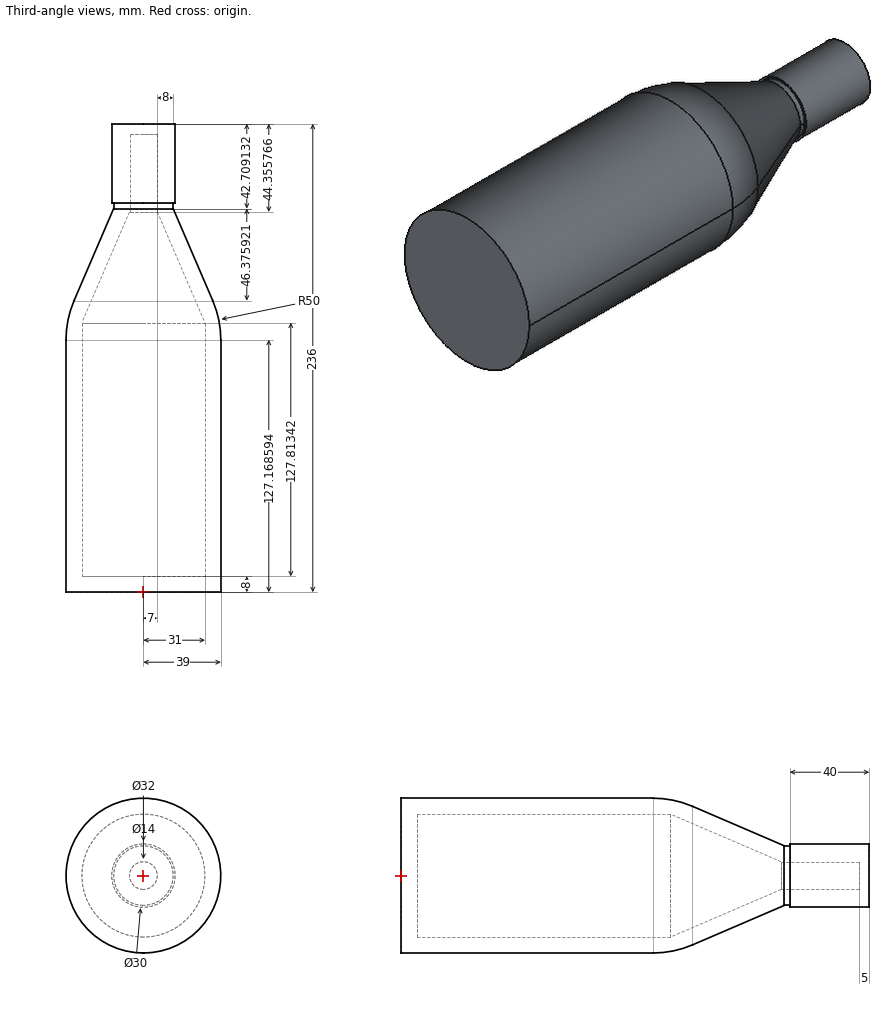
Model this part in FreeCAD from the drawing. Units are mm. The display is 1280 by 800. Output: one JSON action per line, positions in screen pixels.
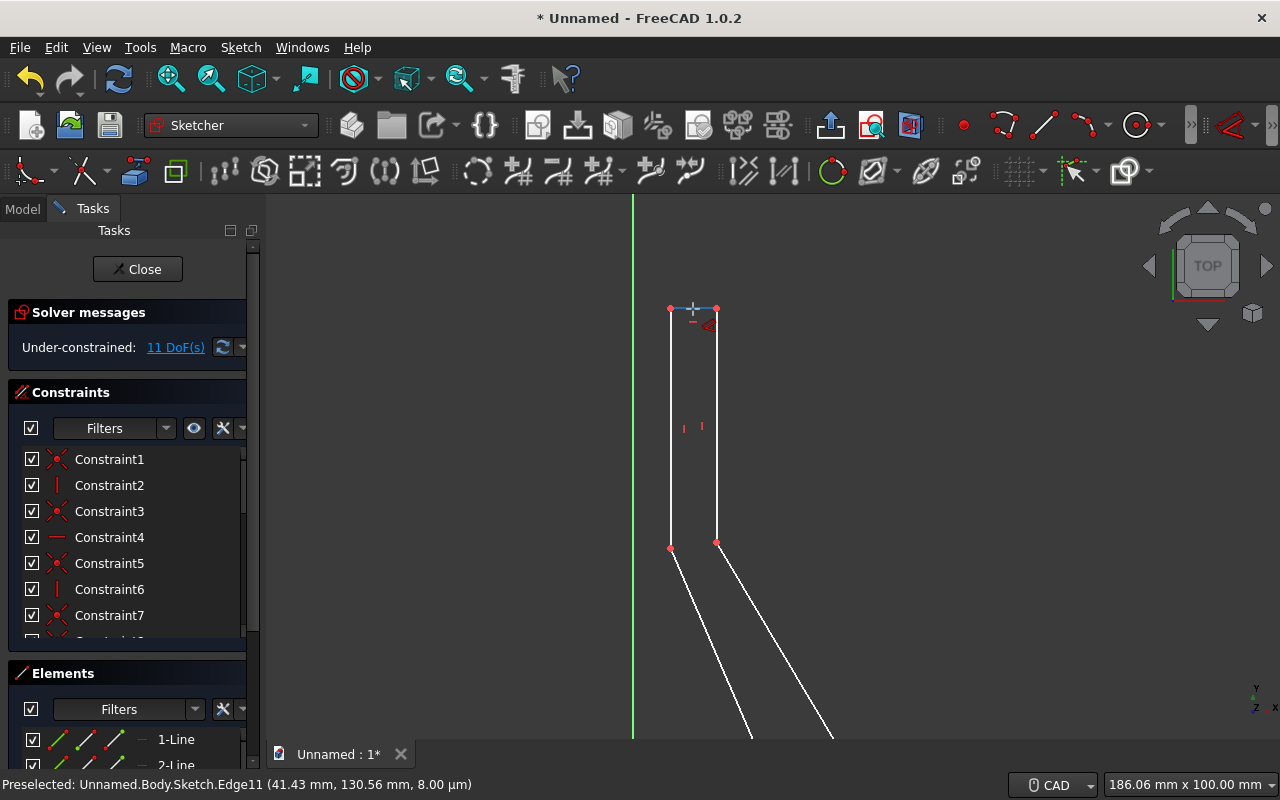
{"action": "left_click", "coordinate": [694, 308]}
{"action": "left_click", "coordinate": [694, 274]}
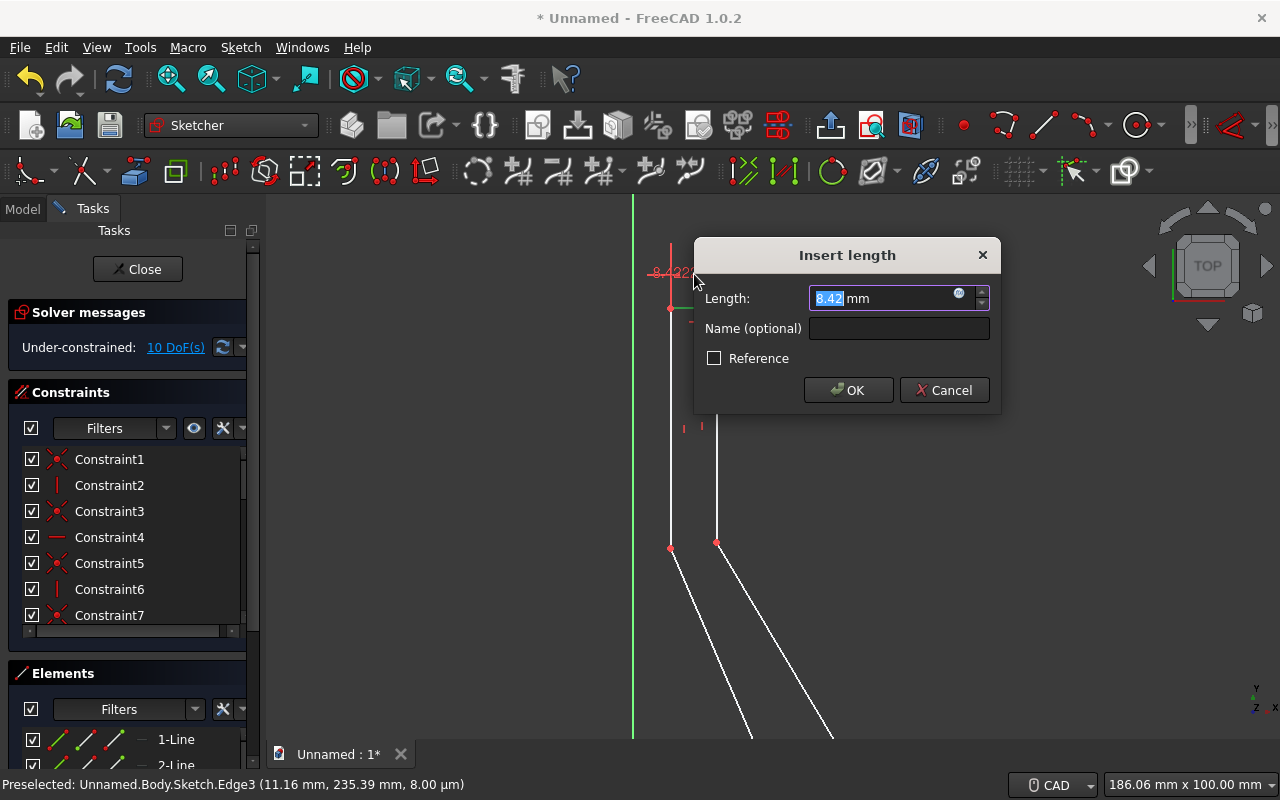
{"action": "type", "text": "8"}
{"action": "key", "text": "Return"}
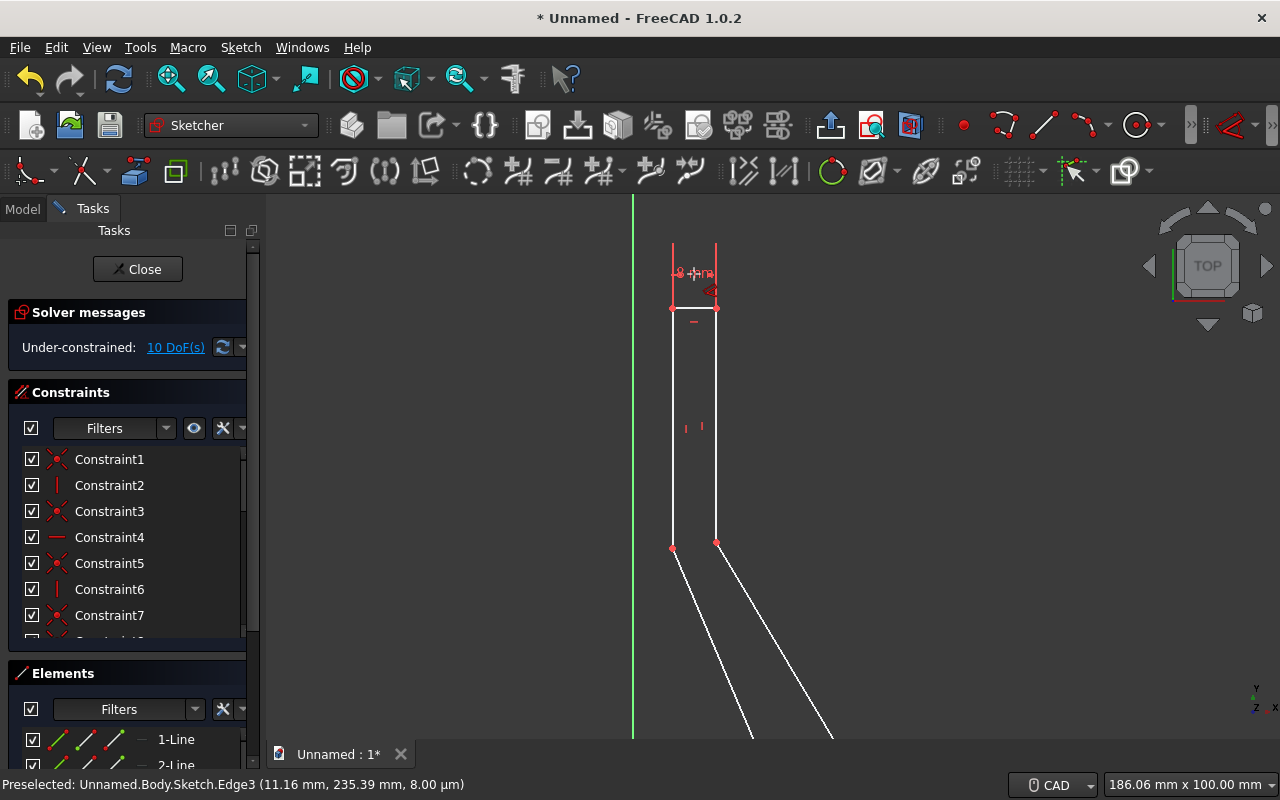
{"action": "scroll", "coordinate": [693, 309], "scroll_direction": "down", "scroll_amount": 7}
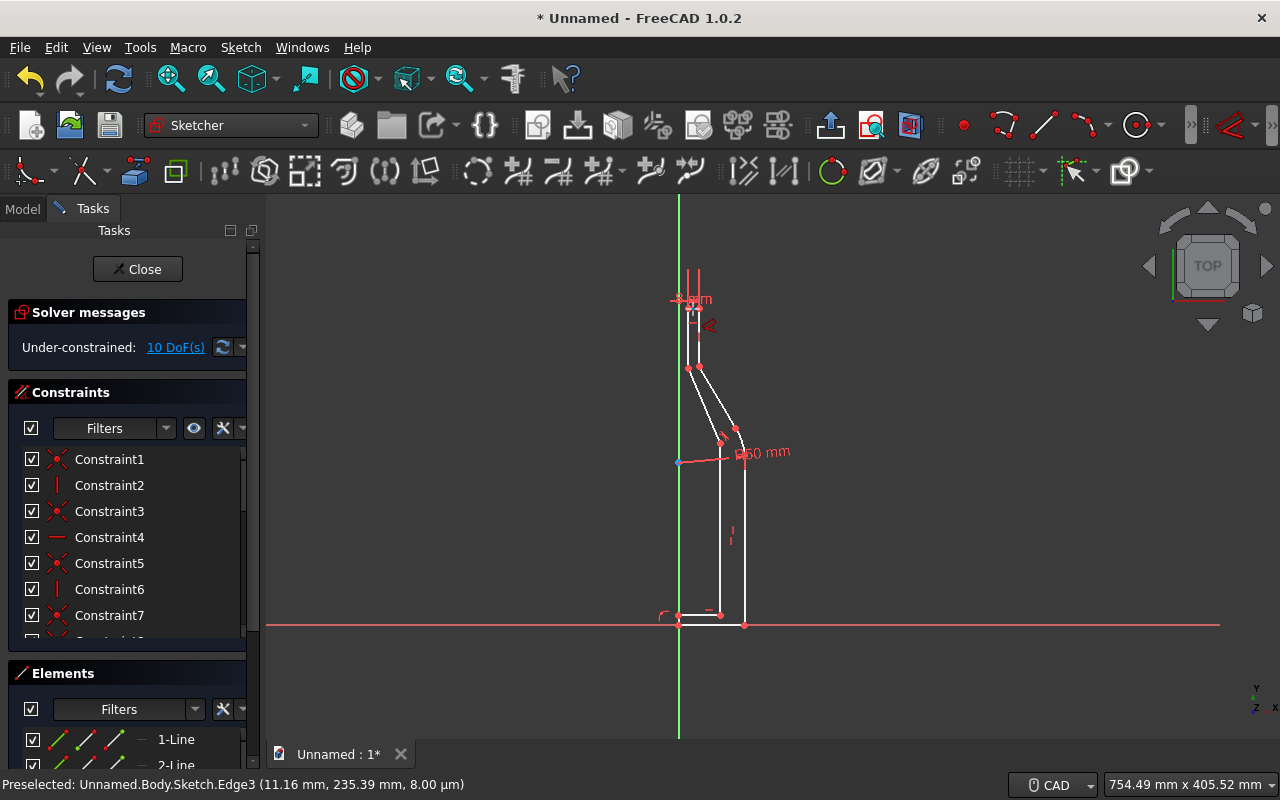
{"action": "scroll", "coordinate": [679, 618], "scroll_direction": "up", "scroll_amount": 8}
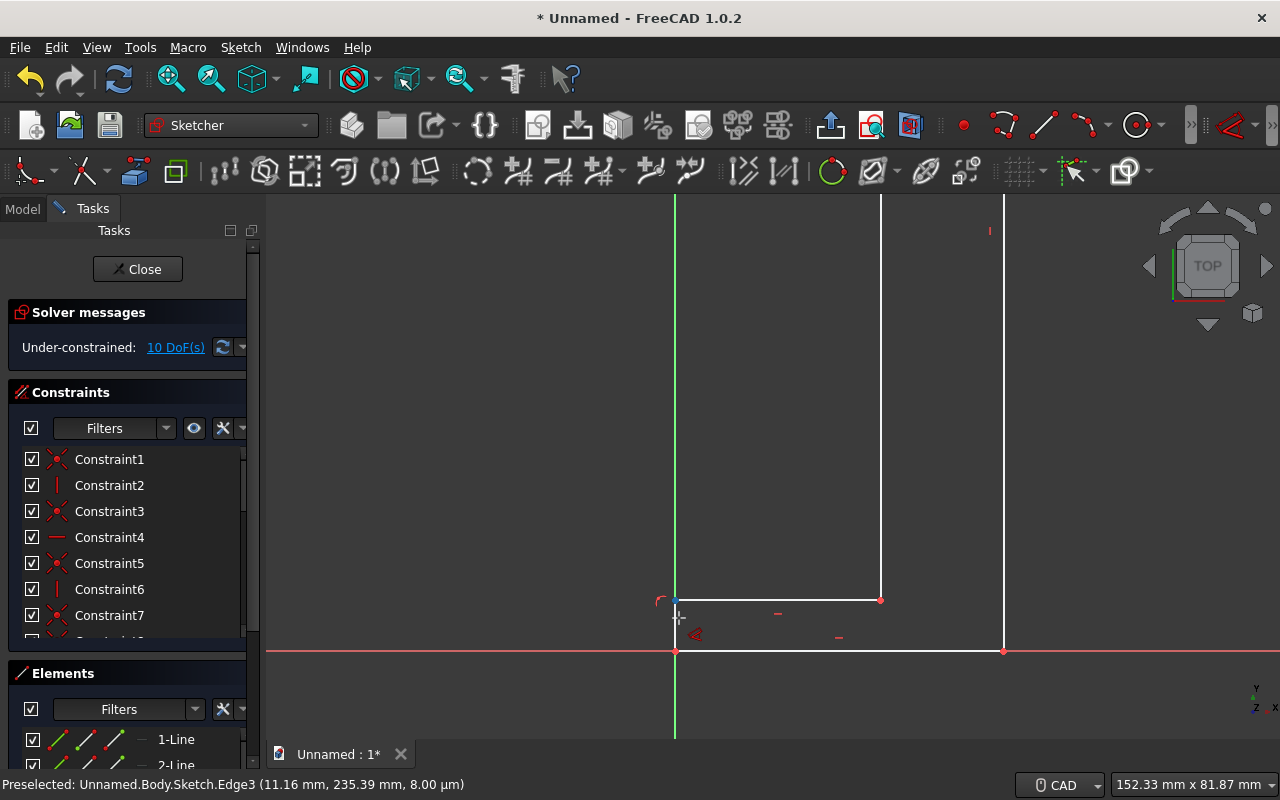
{"action": "left_click", "coordinate": [675, 615]}
{"action": "left_click", "coordinate": [641, 626]}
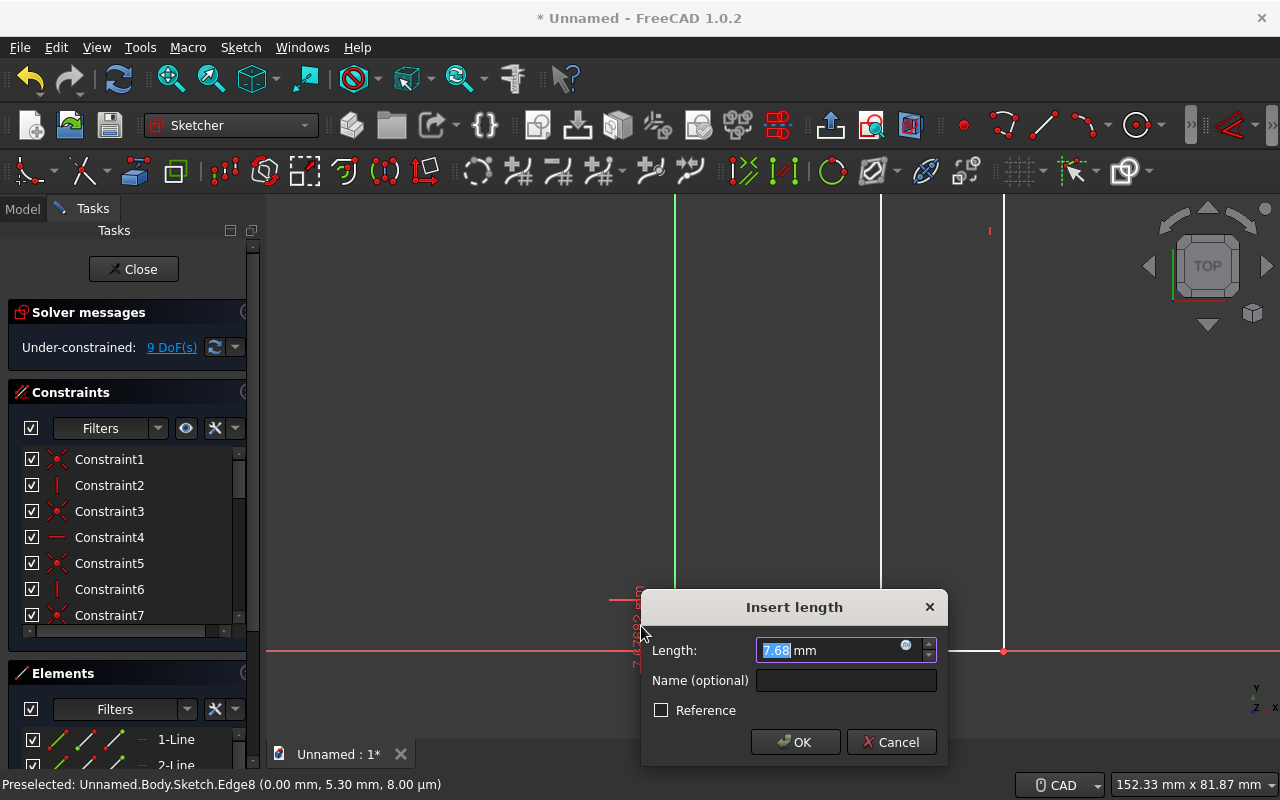
{"action": "type", "text": "8"}
{"action": "key", "text": "Return"}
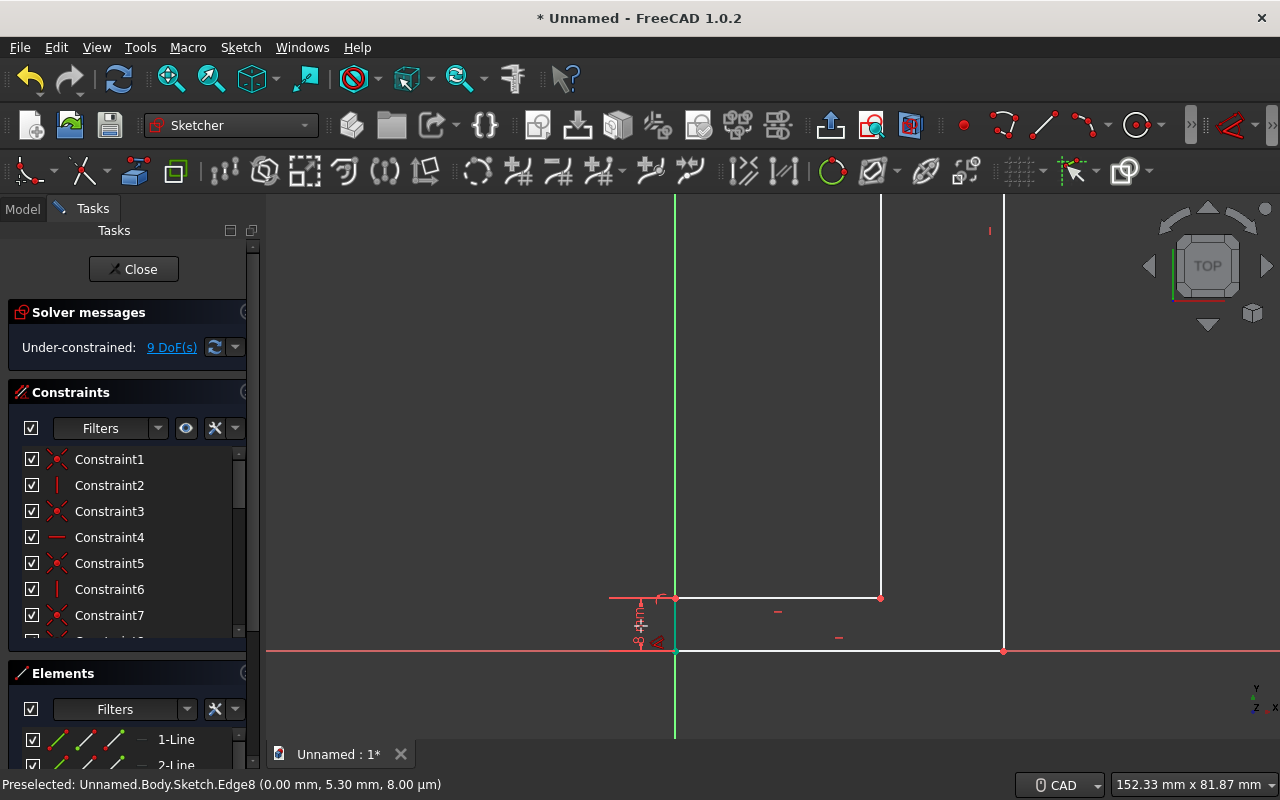
{"action": "scroll", "coordinate": [679, 618], "scroll_direction": "down", "scroll_amount": 8}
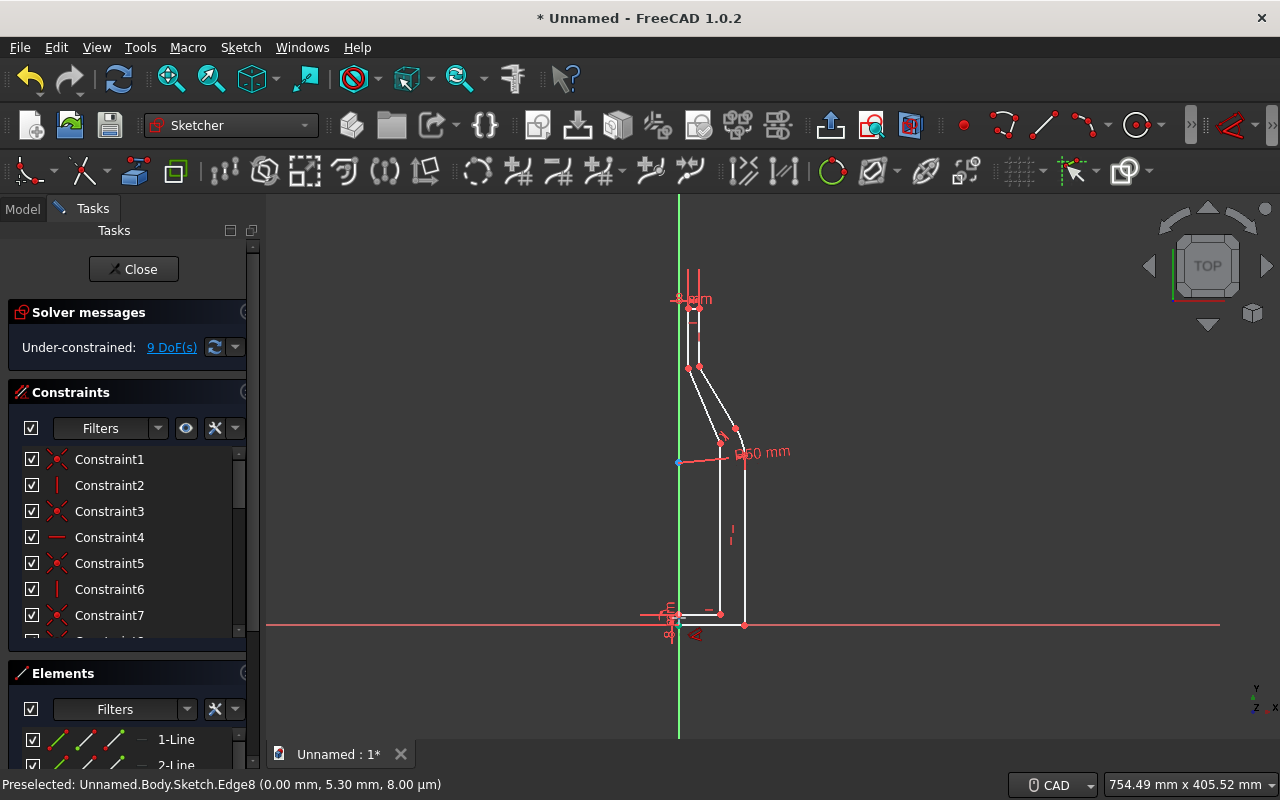
{"action": "scroll", "coordinate": [708, 615], "scroll_direction": "up", "scroll_amount": 2}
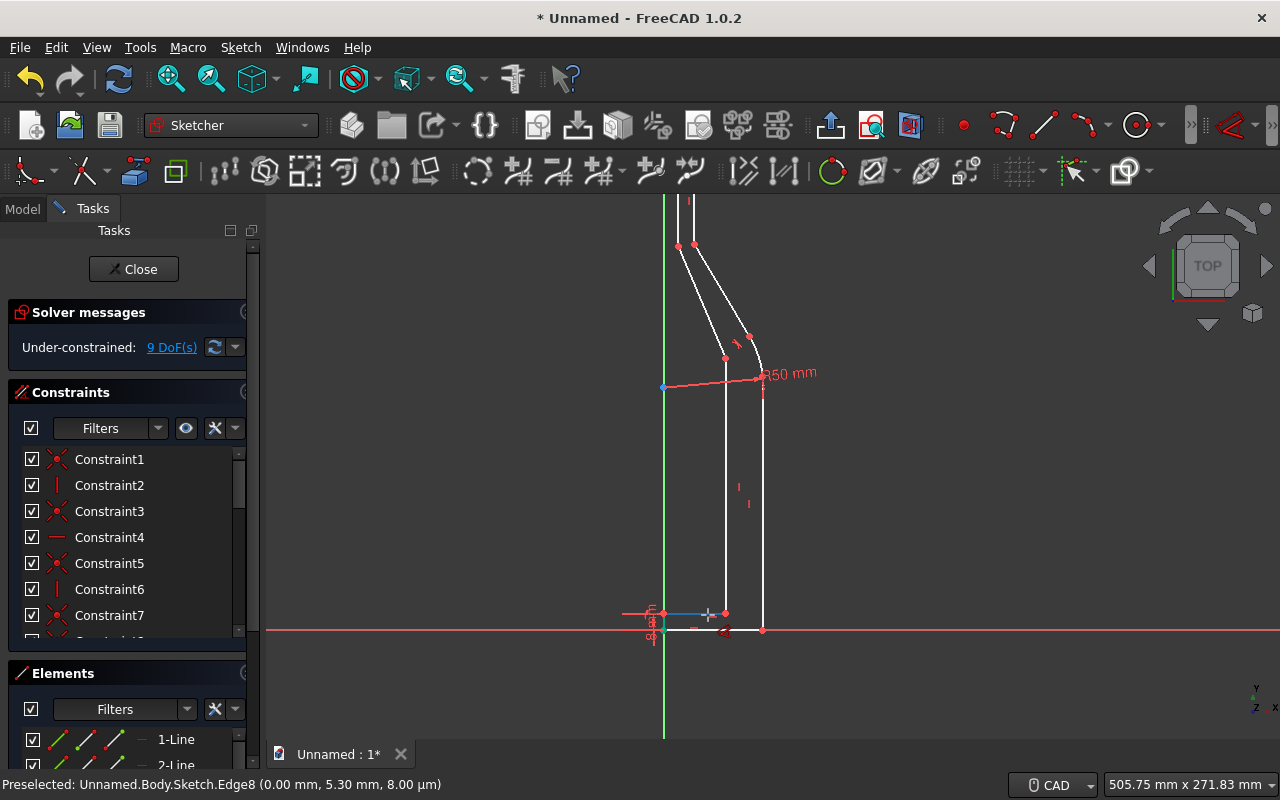
{"action": "left_click", "coordinate": [707, 614]}
{"action": "left_click", "coordinate": [695, 648]}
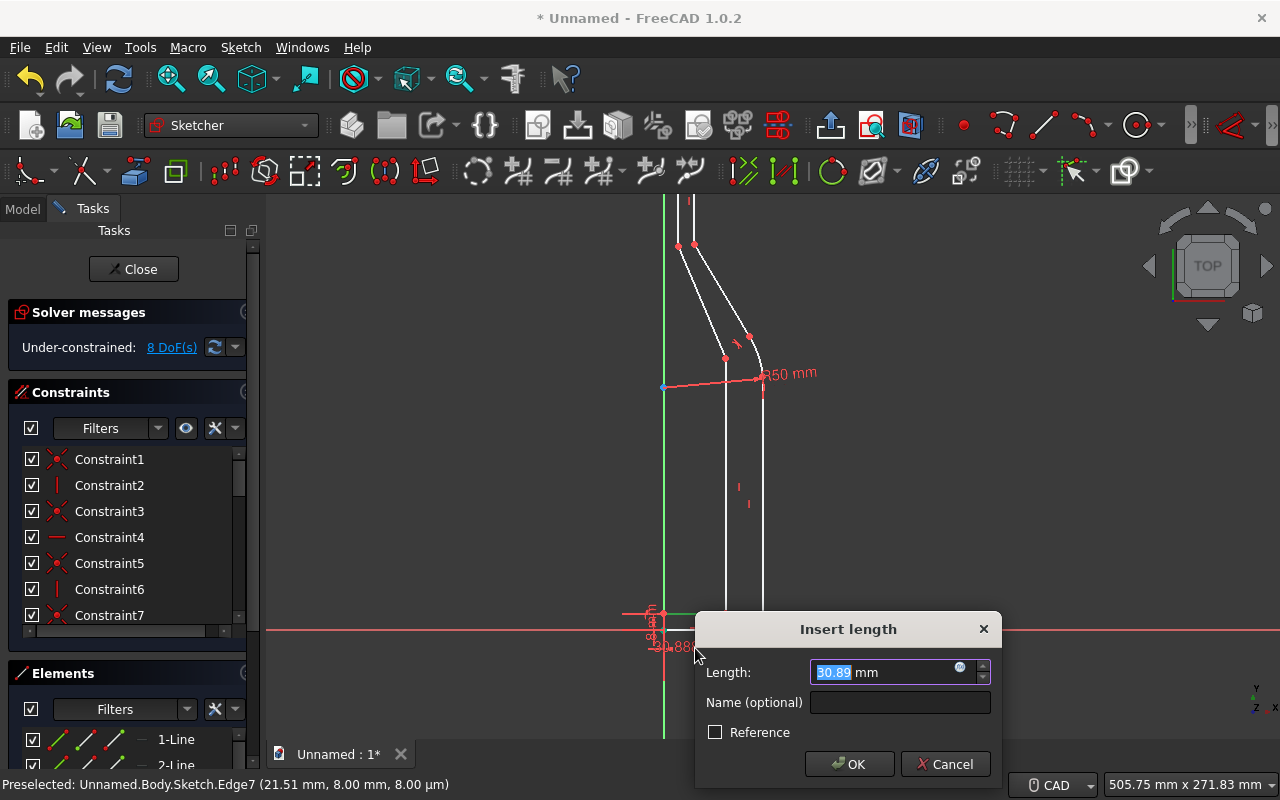
{"action": "type", "text": "31"}
{"action": "key", "text": "Return"}